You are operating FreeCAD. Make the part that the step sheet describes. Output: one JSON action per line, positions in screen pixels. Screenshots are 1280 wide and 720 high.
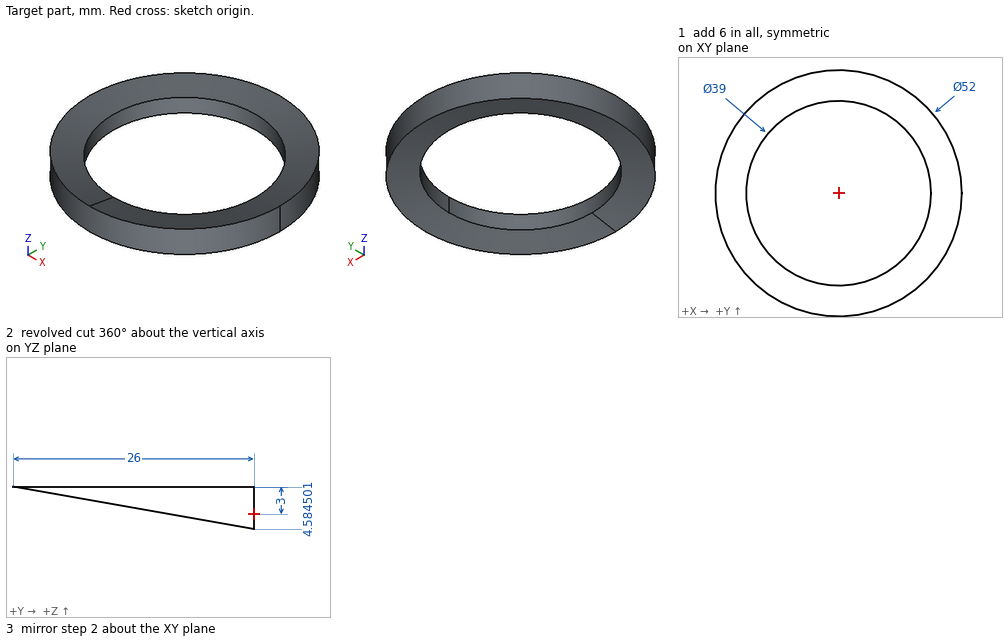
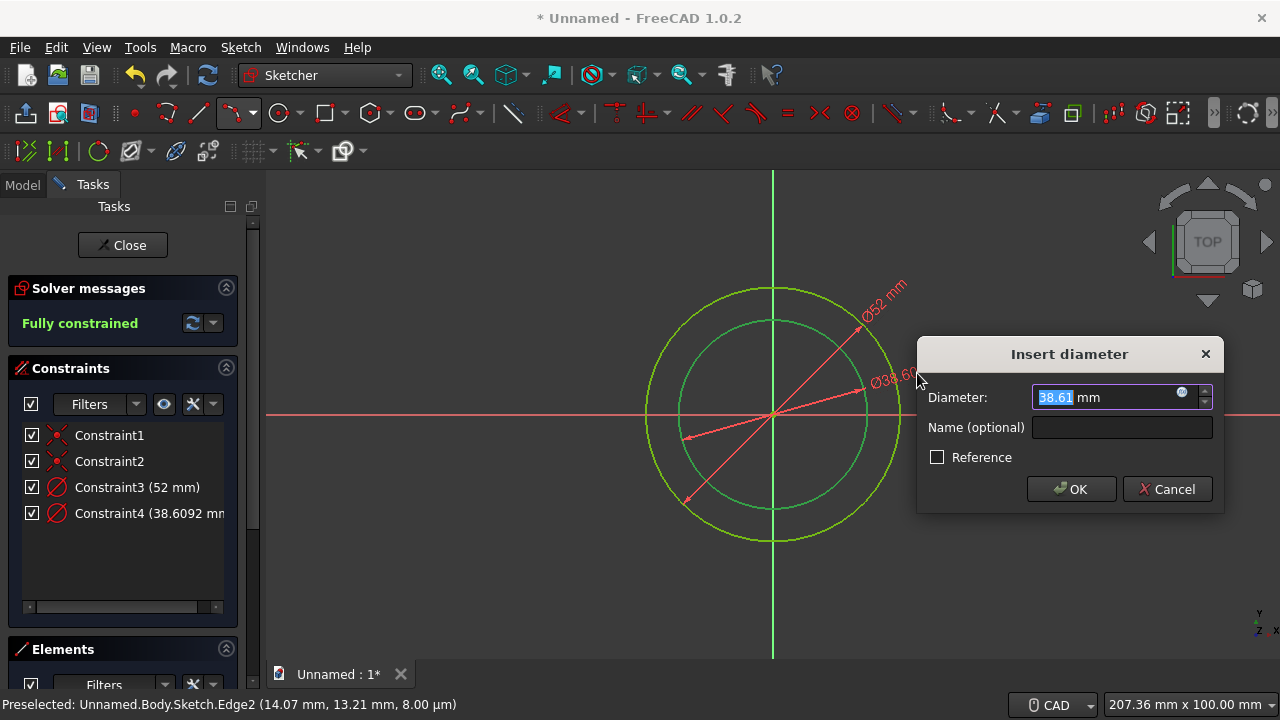
{"action": "type", "text": "39"}
{"action": "key", "text": "Return"}
{"action": "key", "text": "Escape"}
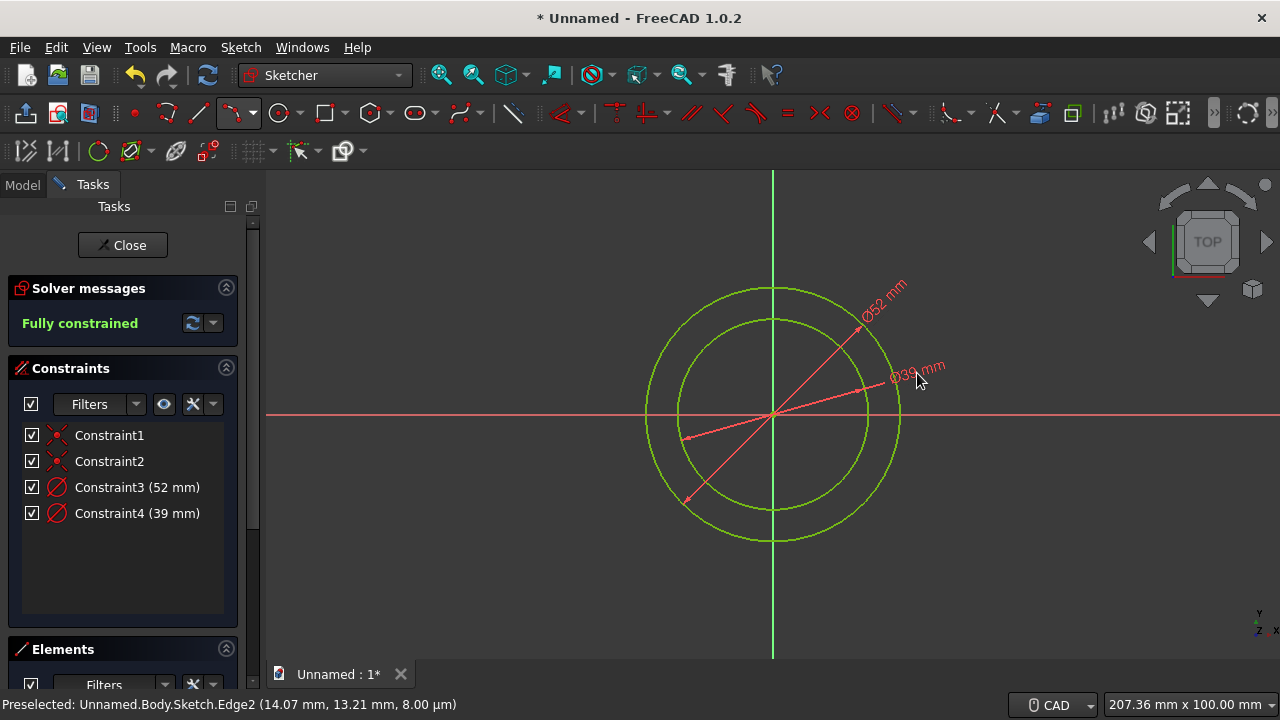
{"action": "left_click", "coordinate": [123, 245]}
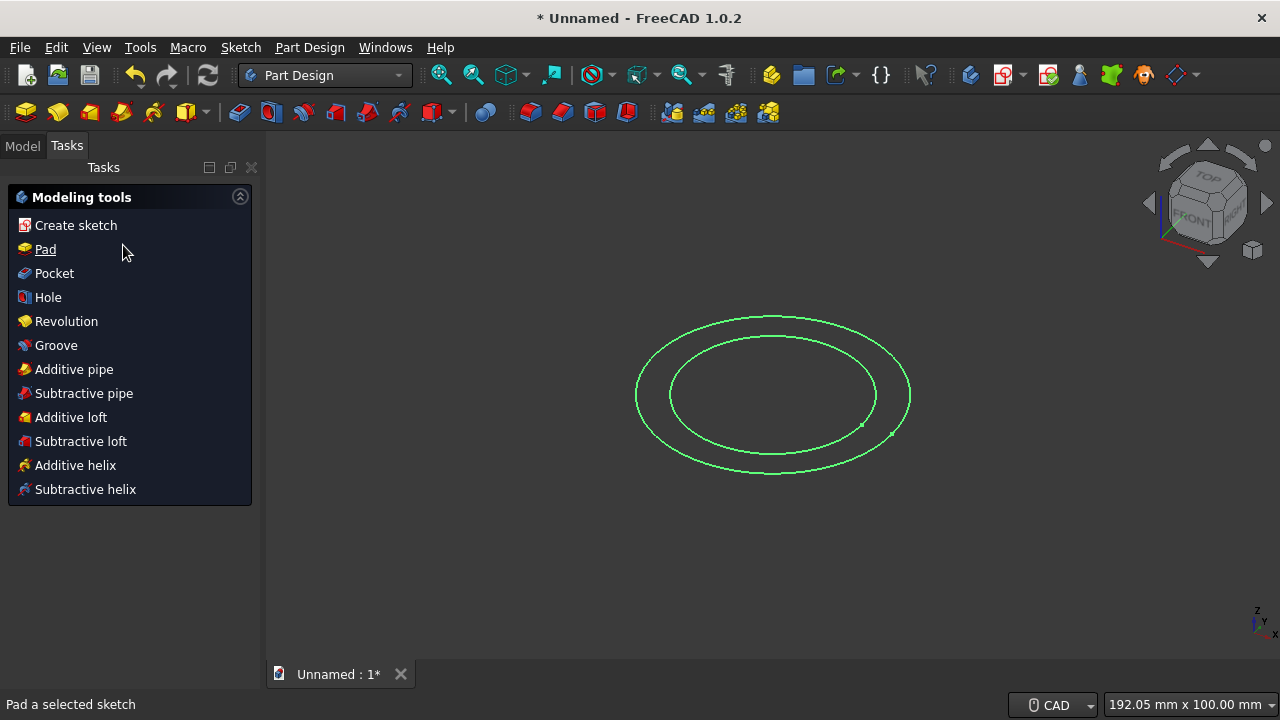
{"action": "left_click", "coordinate": [26, 112]}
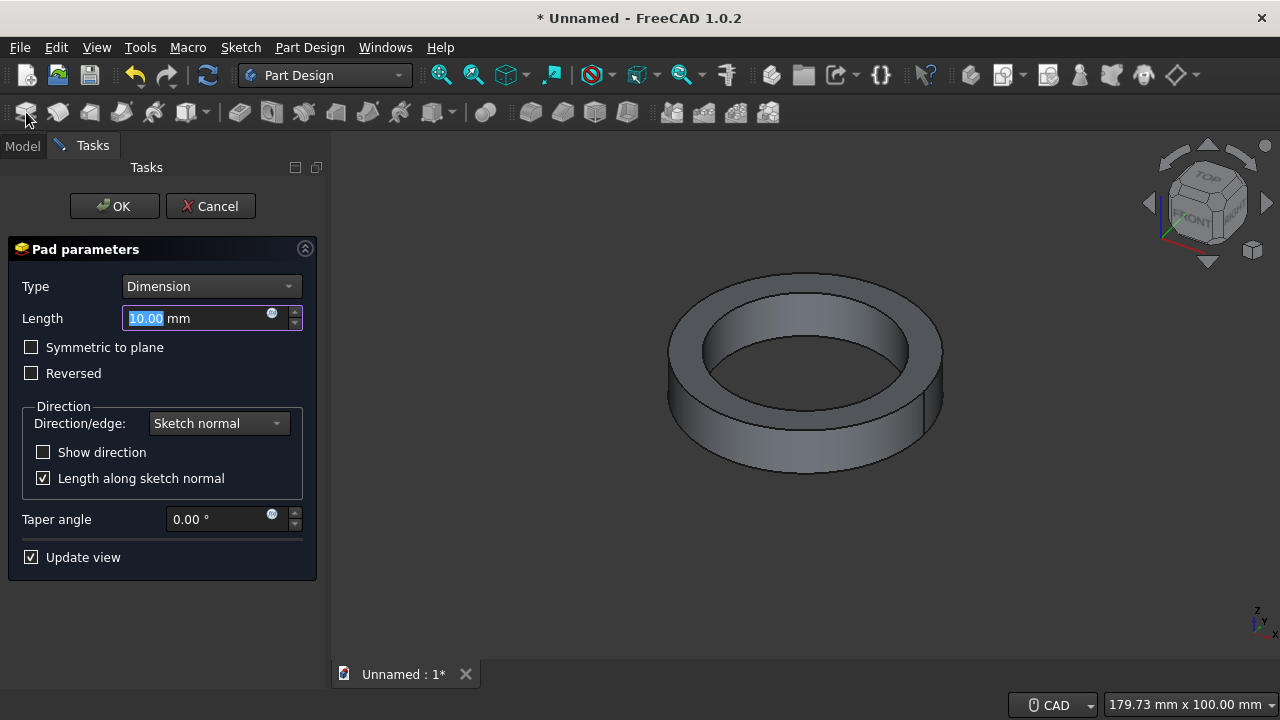
{"action": "type", "text": "6"}
{"action": "key", "text": "Tab"}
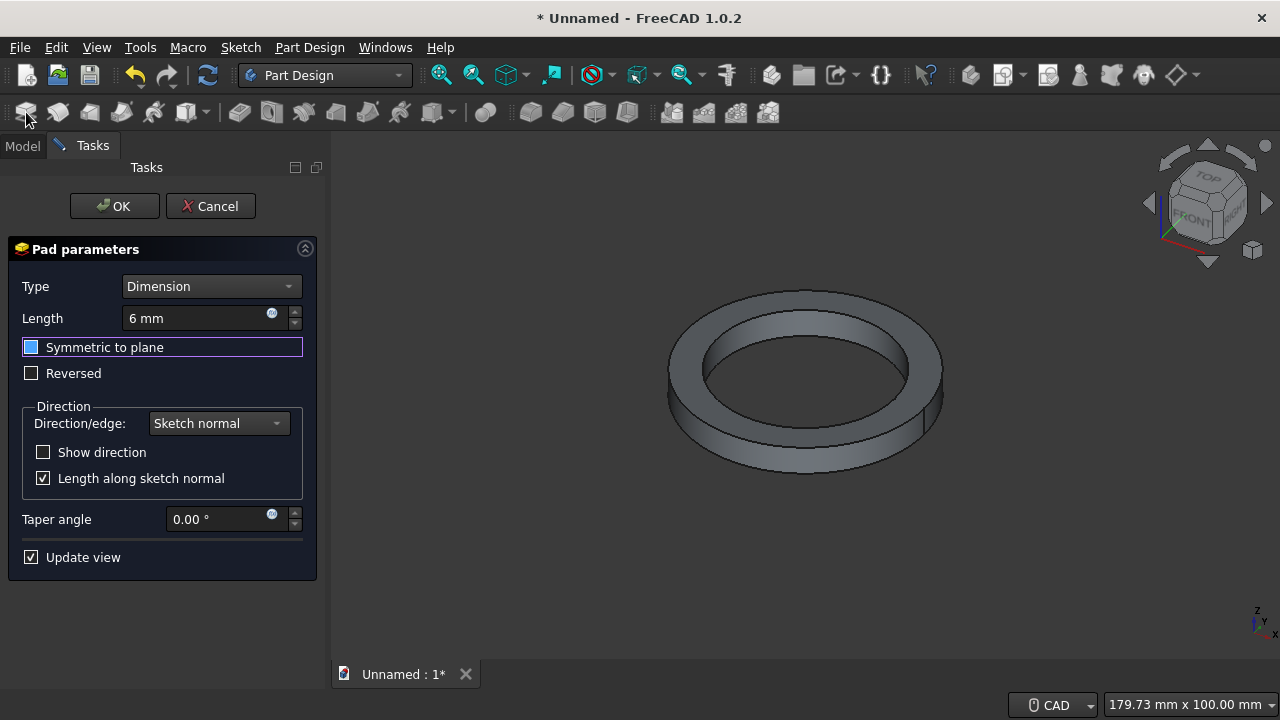
{"action": "left_click", "coordinate": [30, 347]}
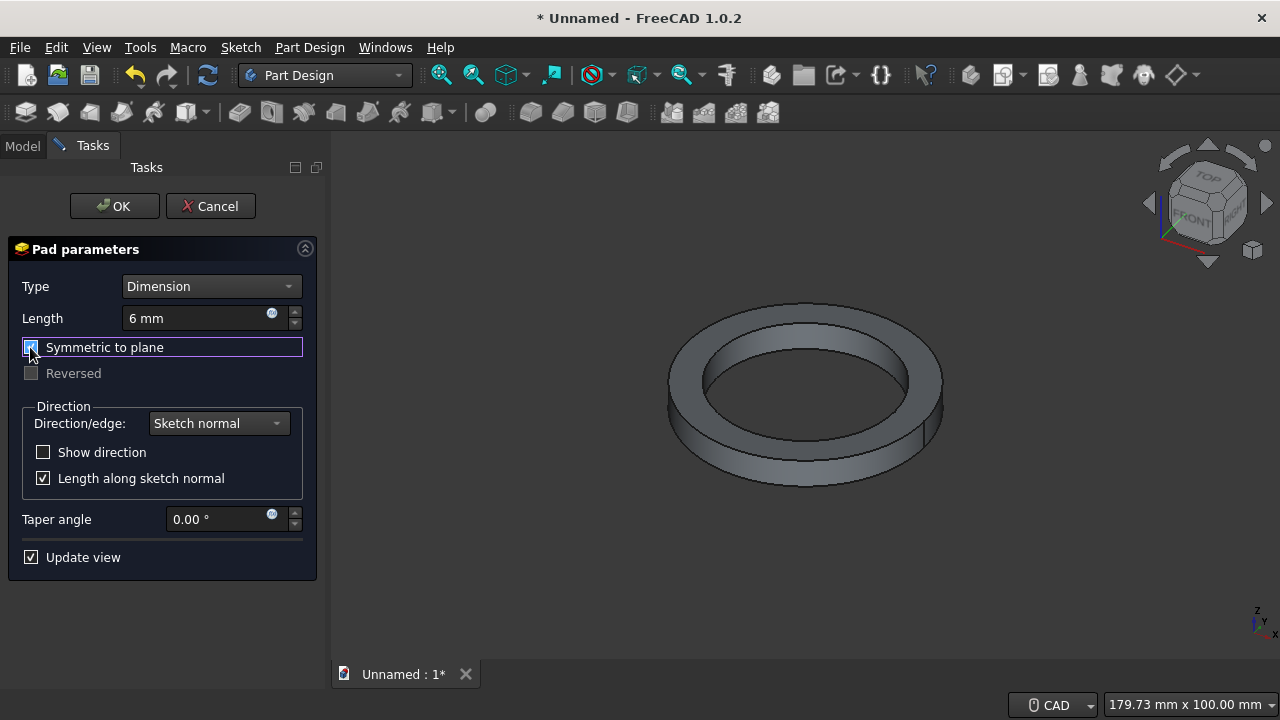
{"action": "left_click", "coordinate": [115, 206]}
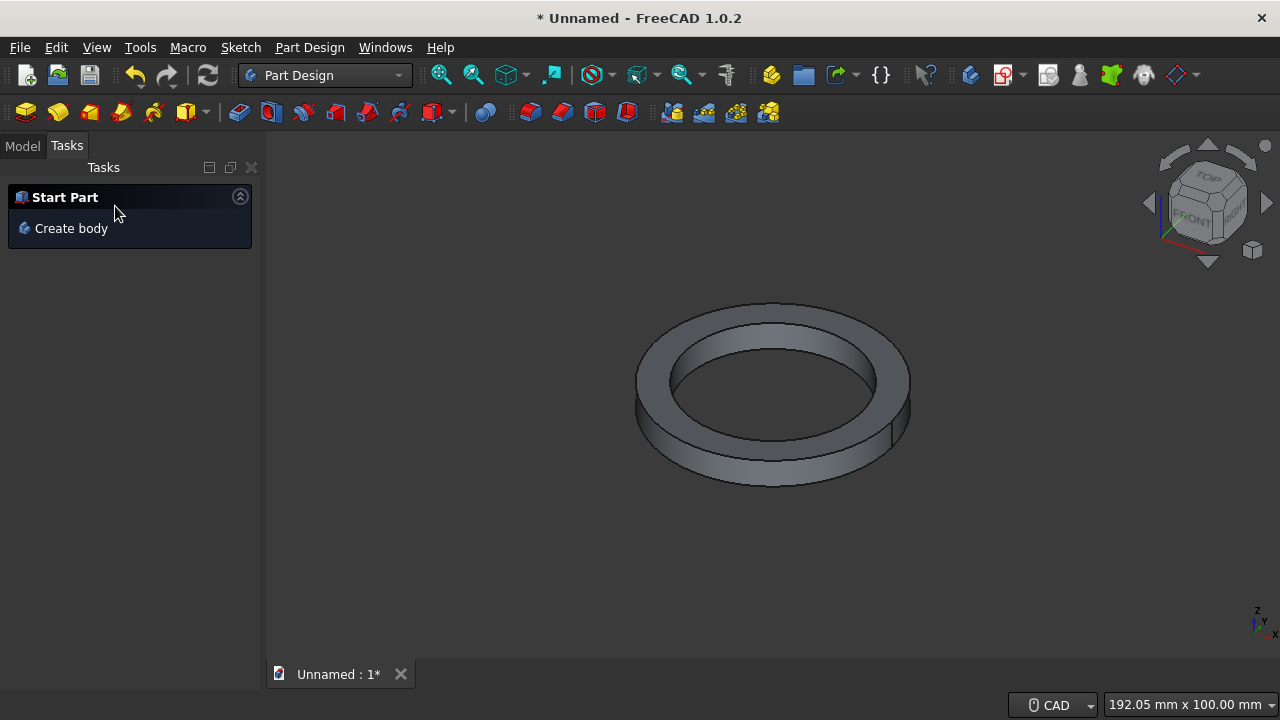
{"action": "left_click", "coordinate": [1004, 76]}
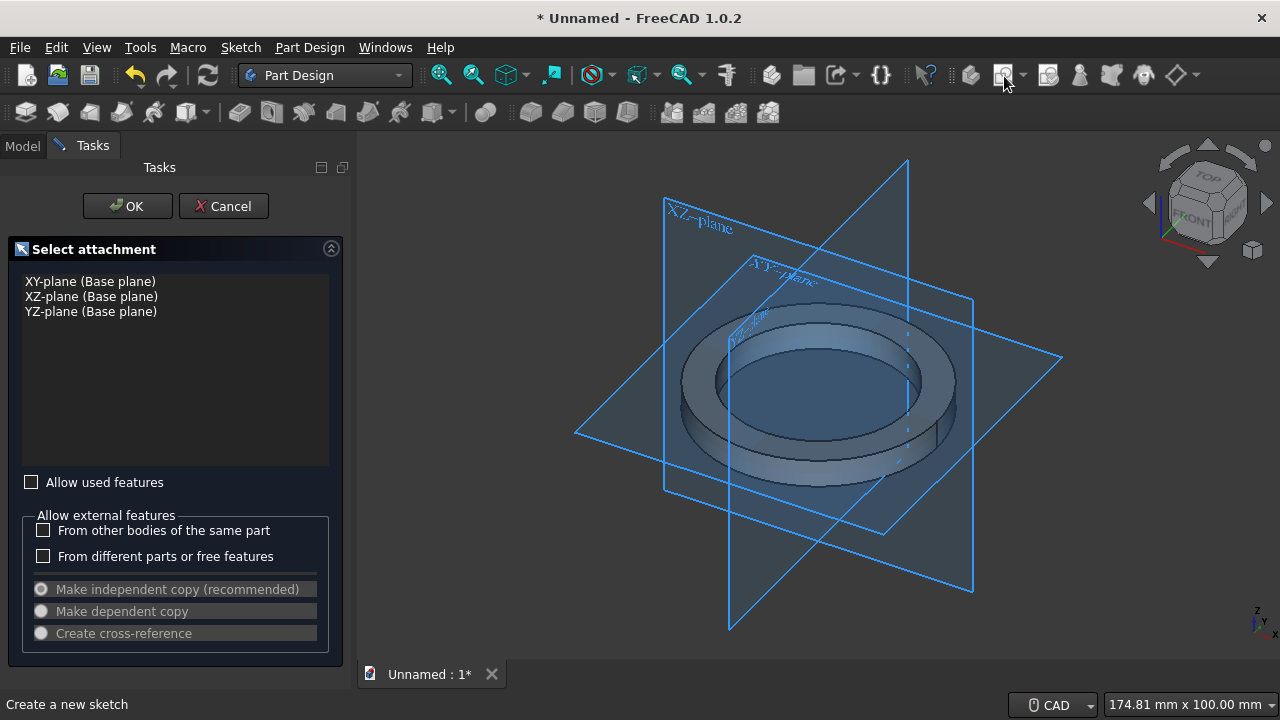
{"action": "left_click", "coordinate": [82, 312]}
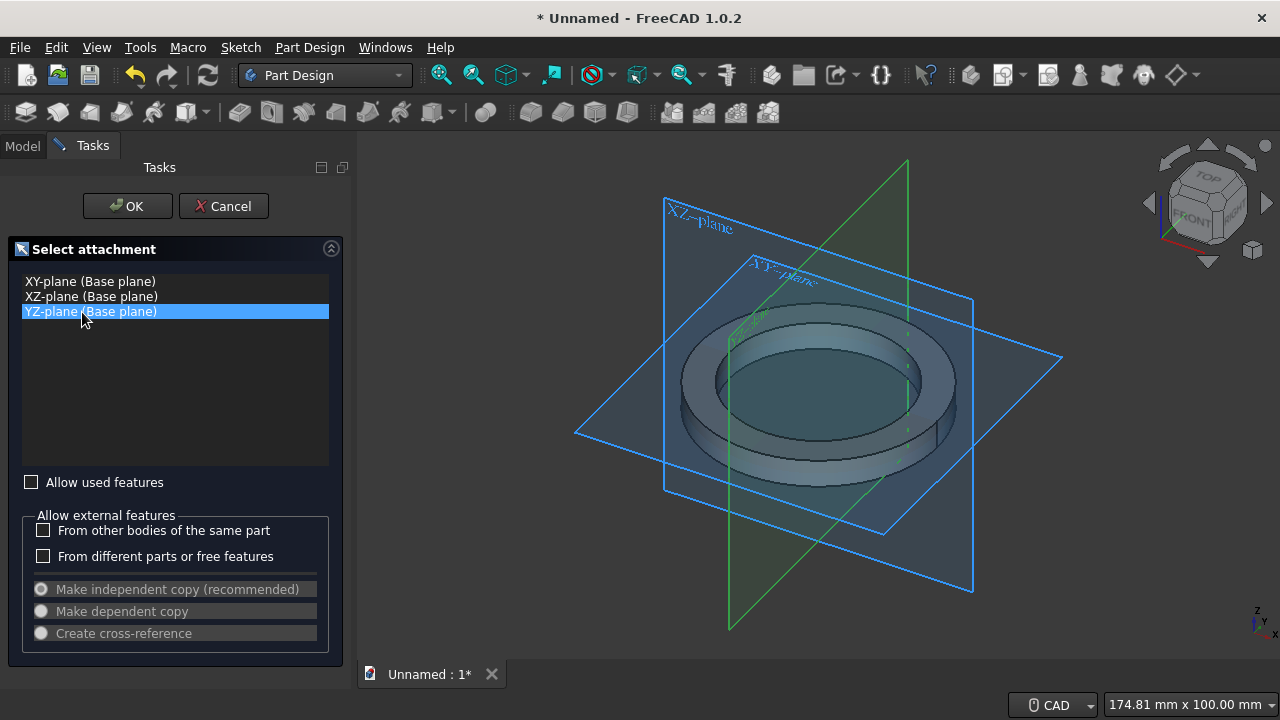
{"action": "left_click", "coordinate": [128, 206]}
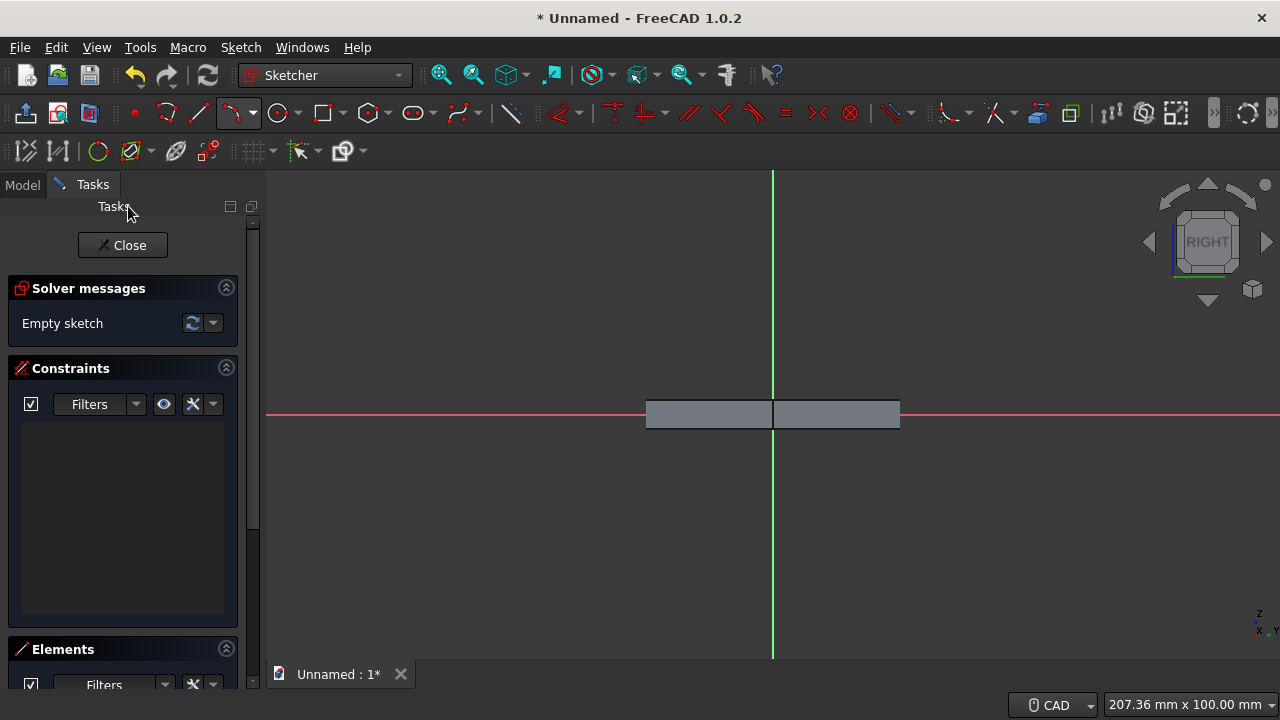
{"action": "key", "text": "q s"}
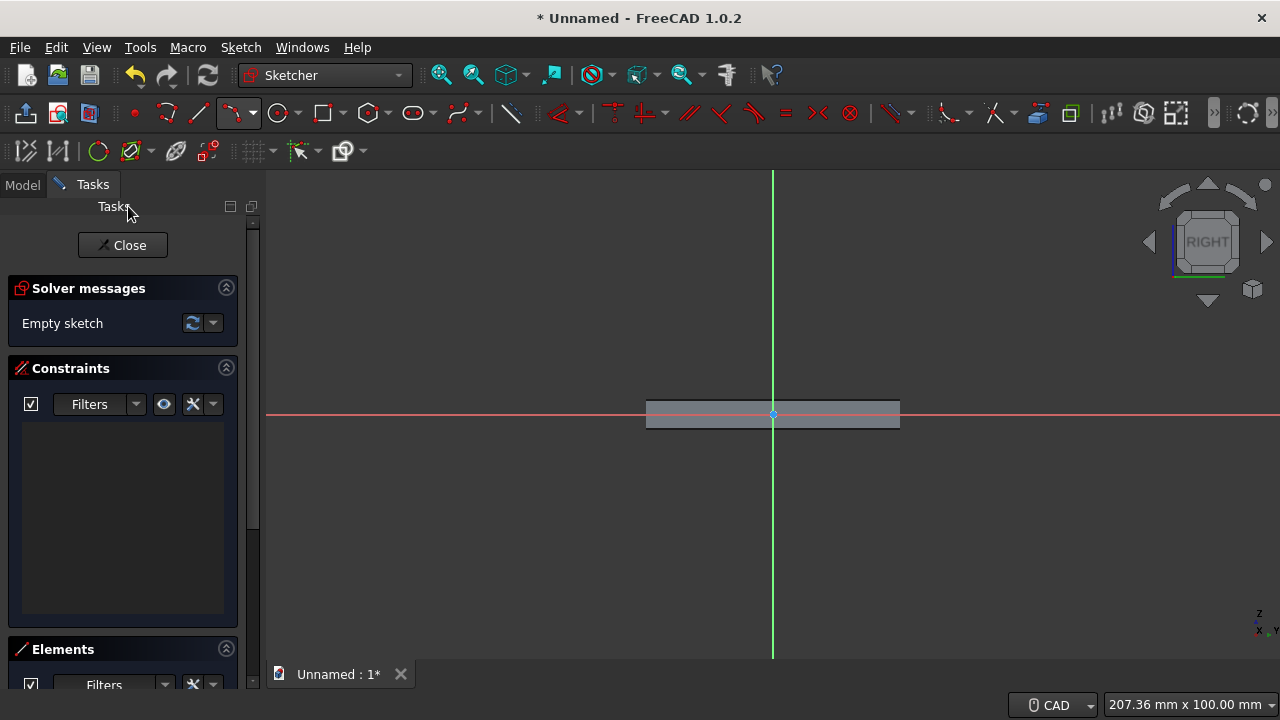
{"action": "scroll", "coordinate": [711, 410], "scroll_direction": "up", "scroll_amount": 8}